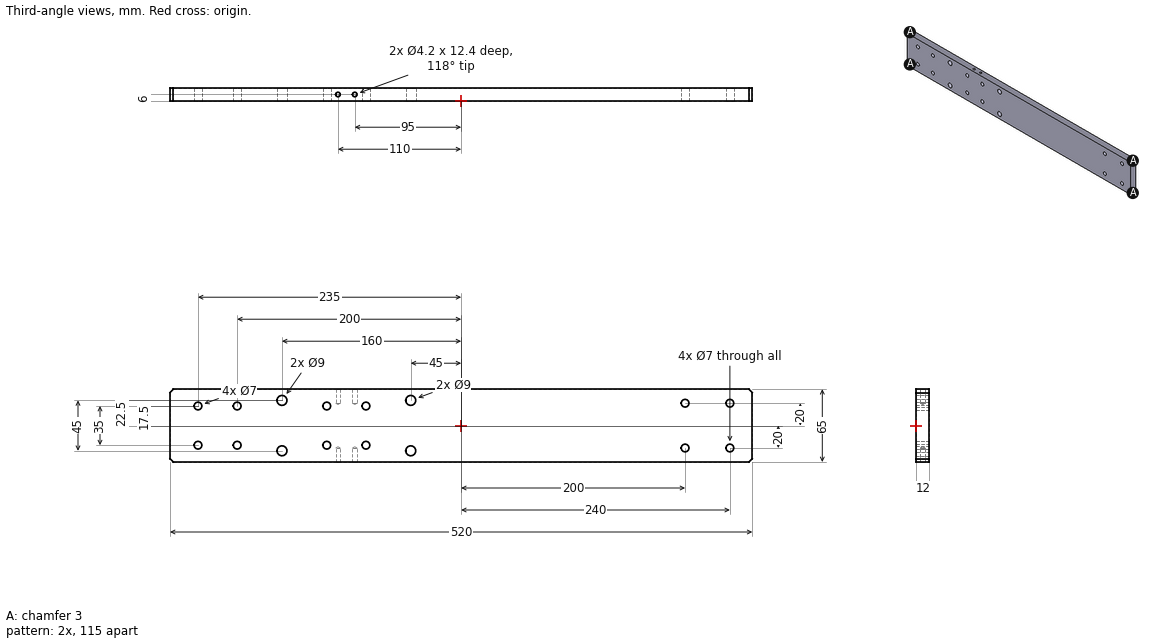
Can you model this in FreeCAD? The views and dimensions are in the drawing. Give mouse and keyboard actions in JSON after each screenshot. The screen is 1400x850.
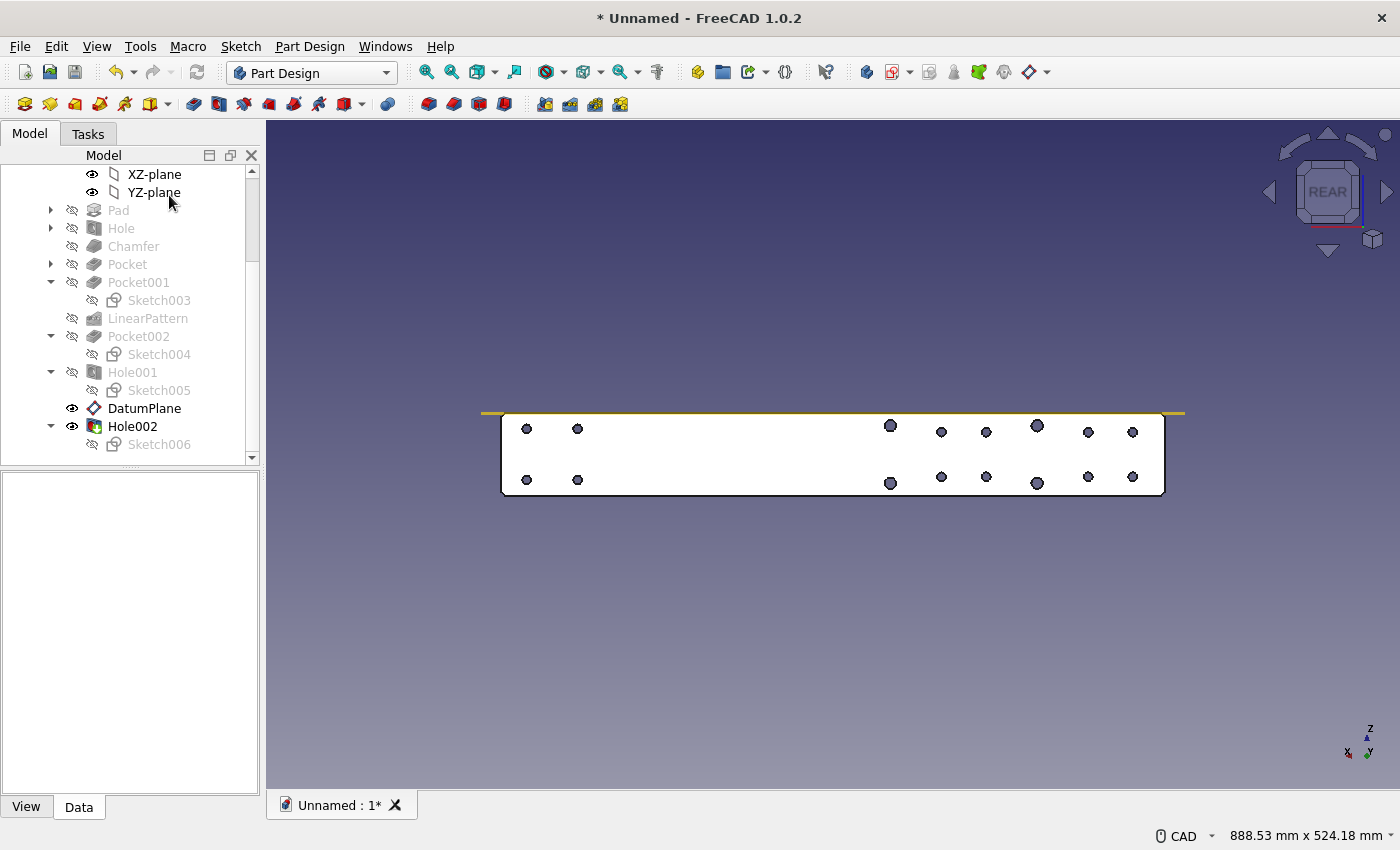
{"action": "left_click", "coordinate": [117, 408]}
{"action": "key", "text": "space"}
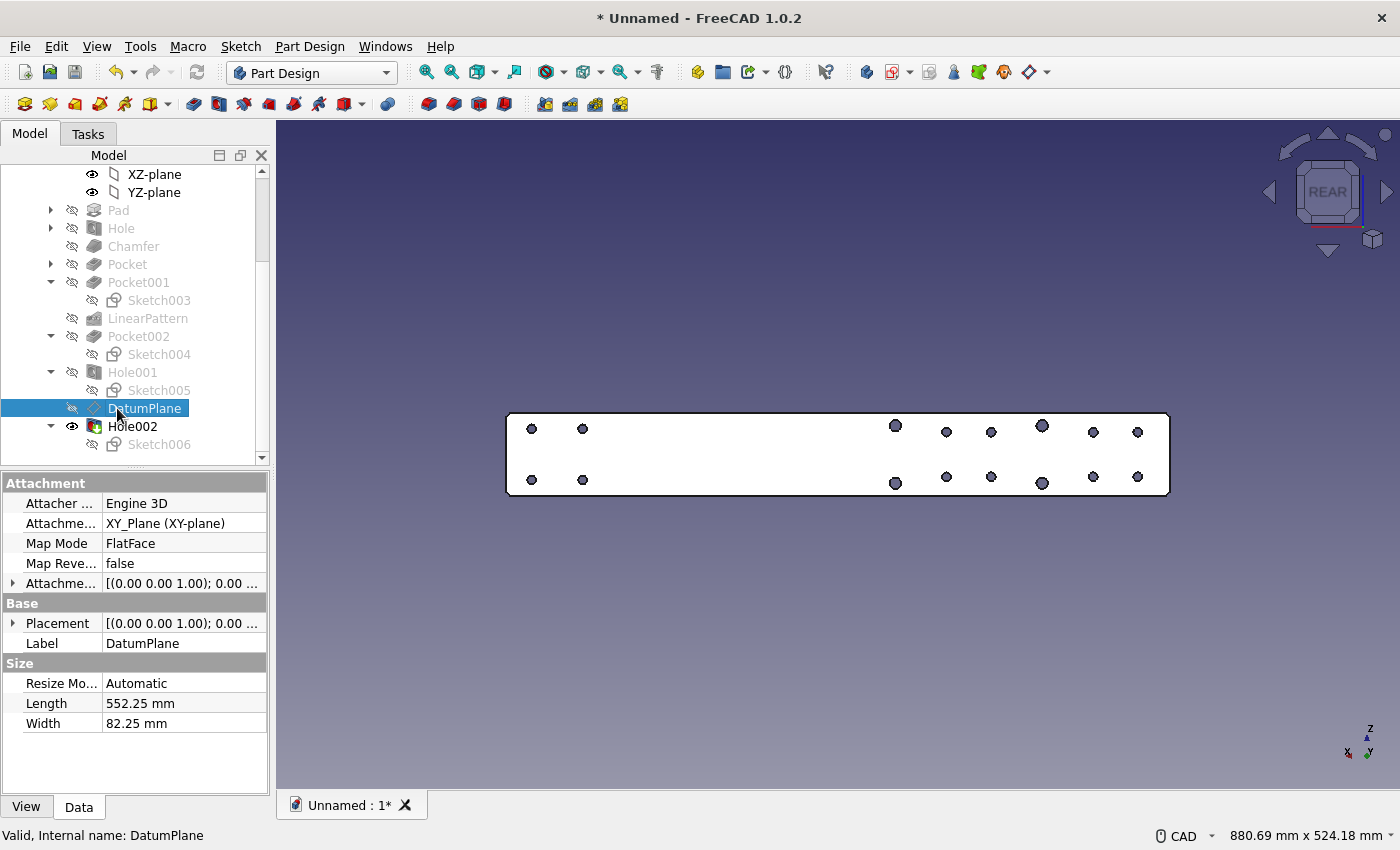
{"action": "key", "text": "0"}